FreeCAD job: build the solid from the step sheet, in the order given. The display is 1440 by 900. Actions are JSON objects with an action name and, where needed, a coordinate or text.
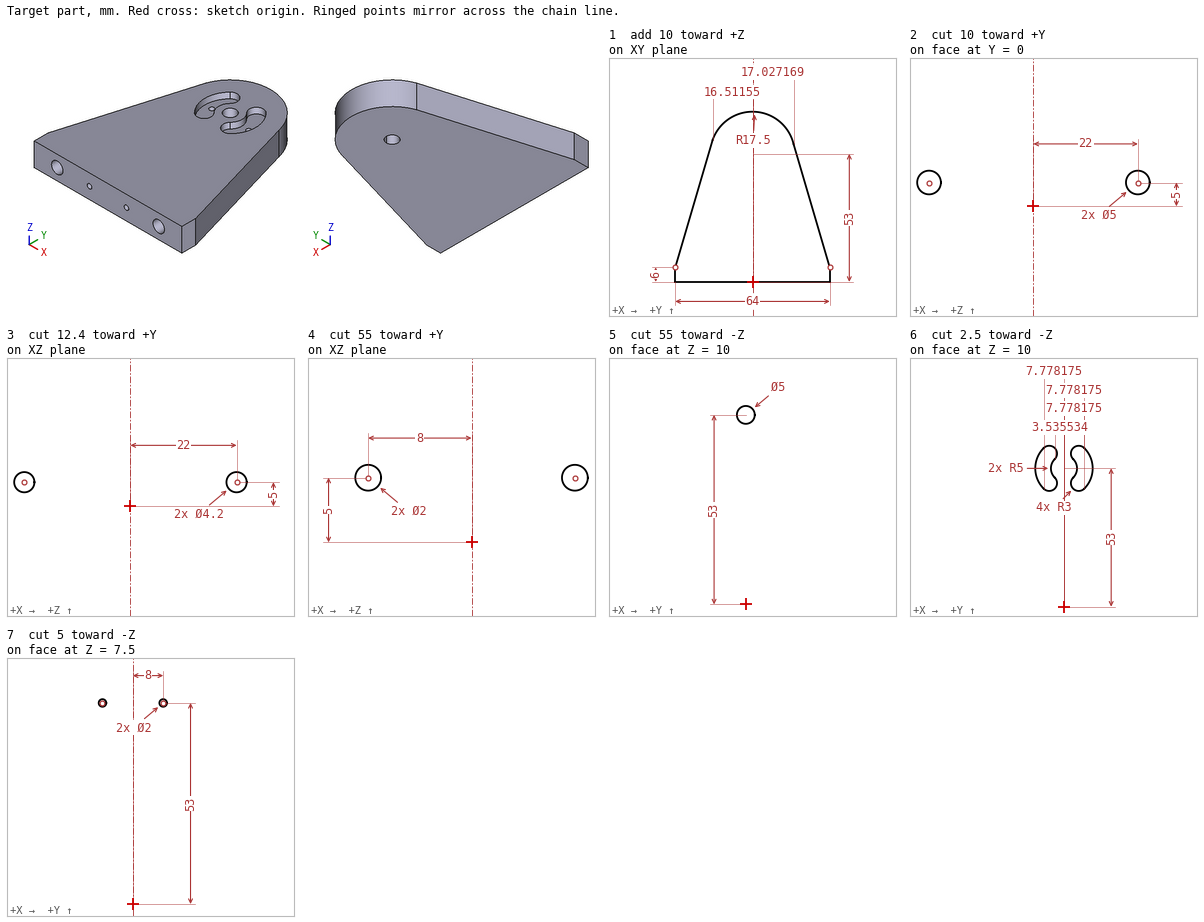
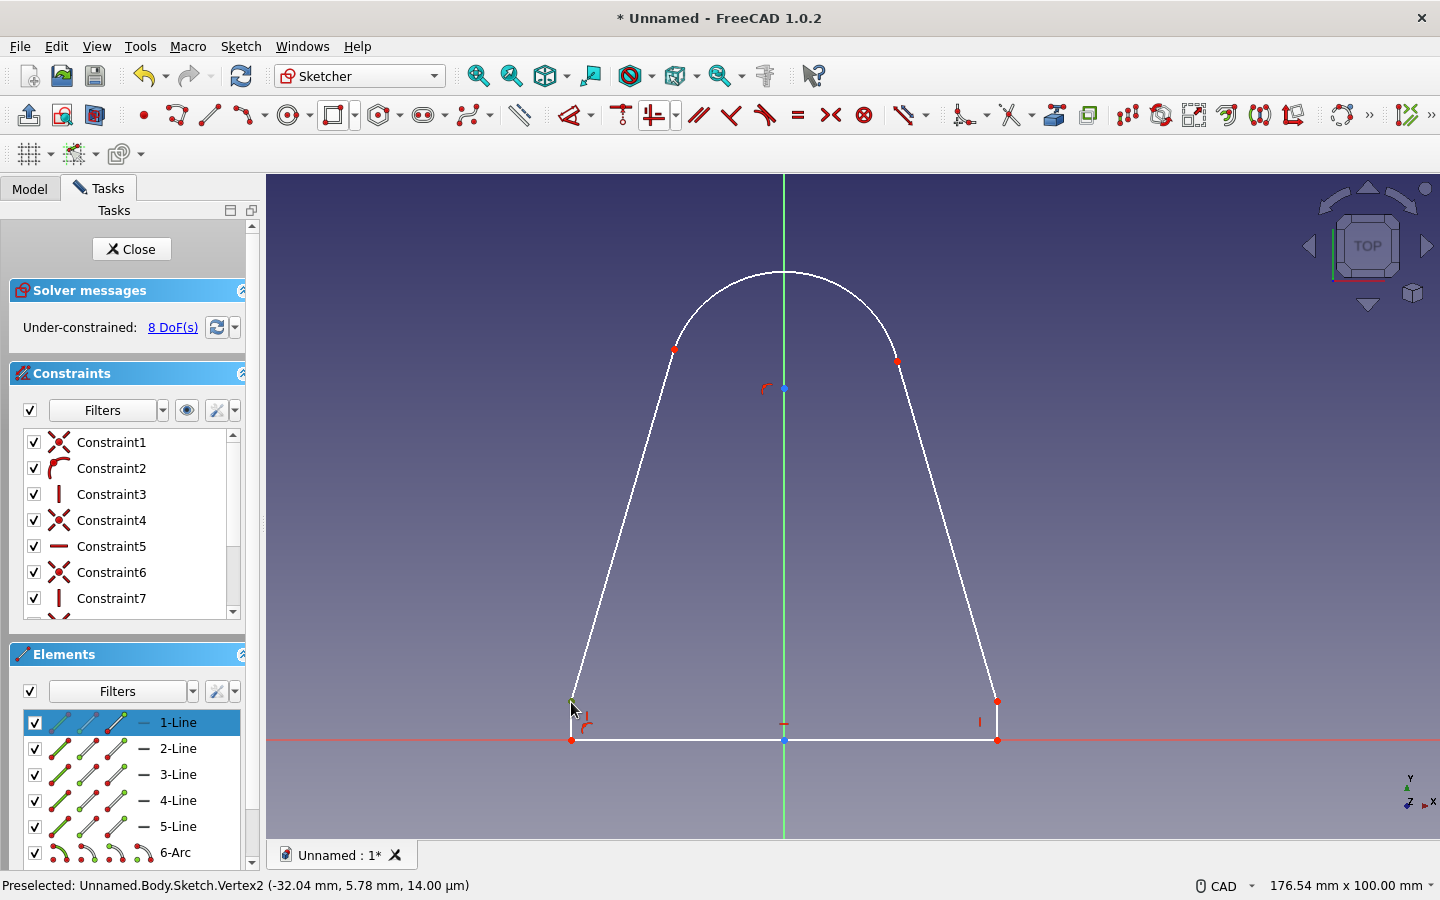
{"action": "left_click", "coordinate": [997, 702]}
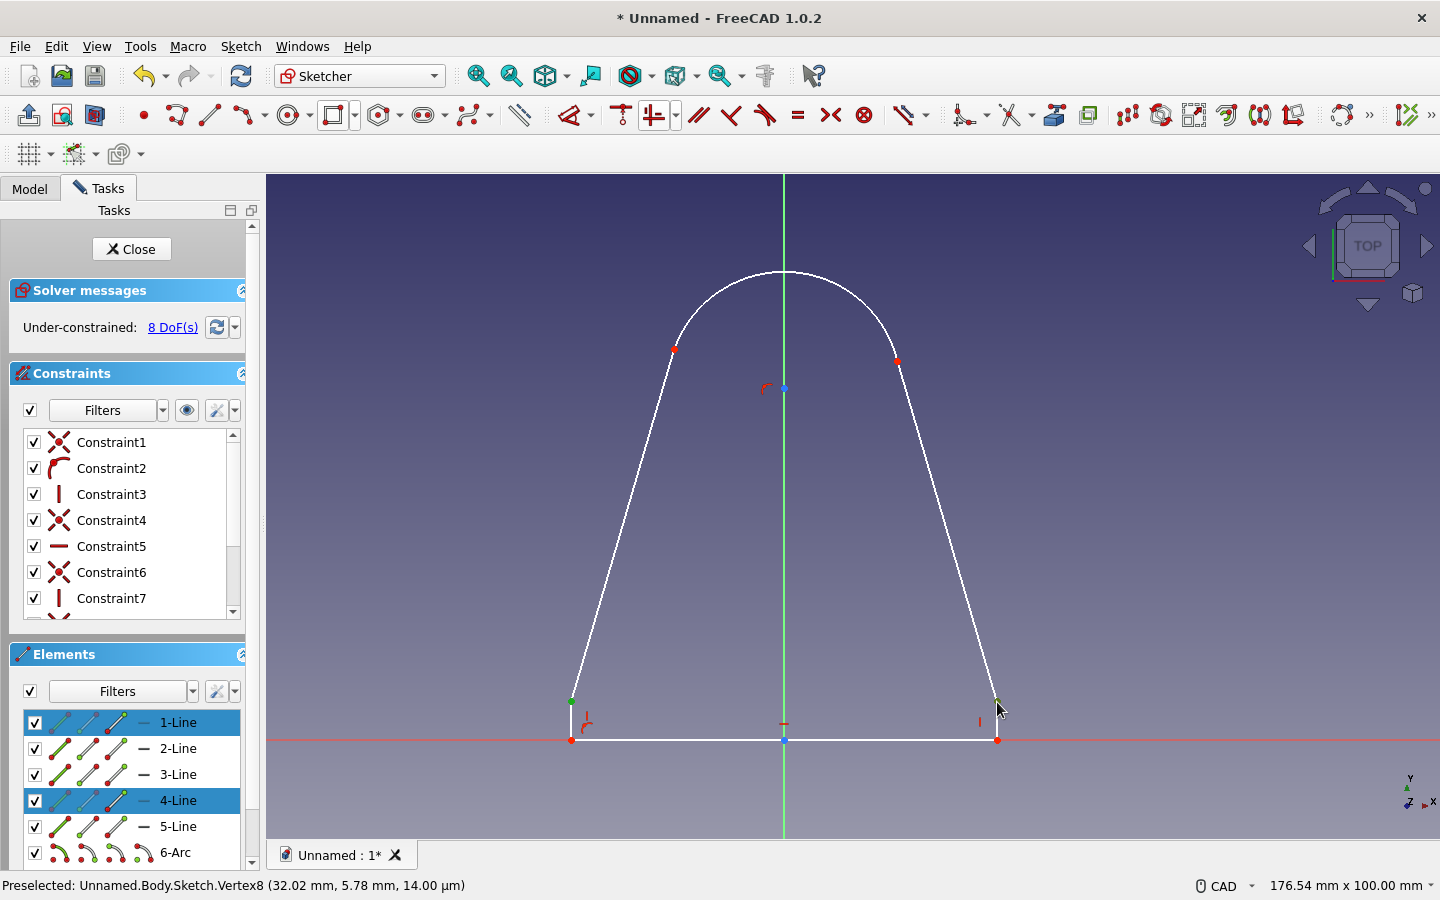
{"action": "left_click", "coordinate": [784, 680]}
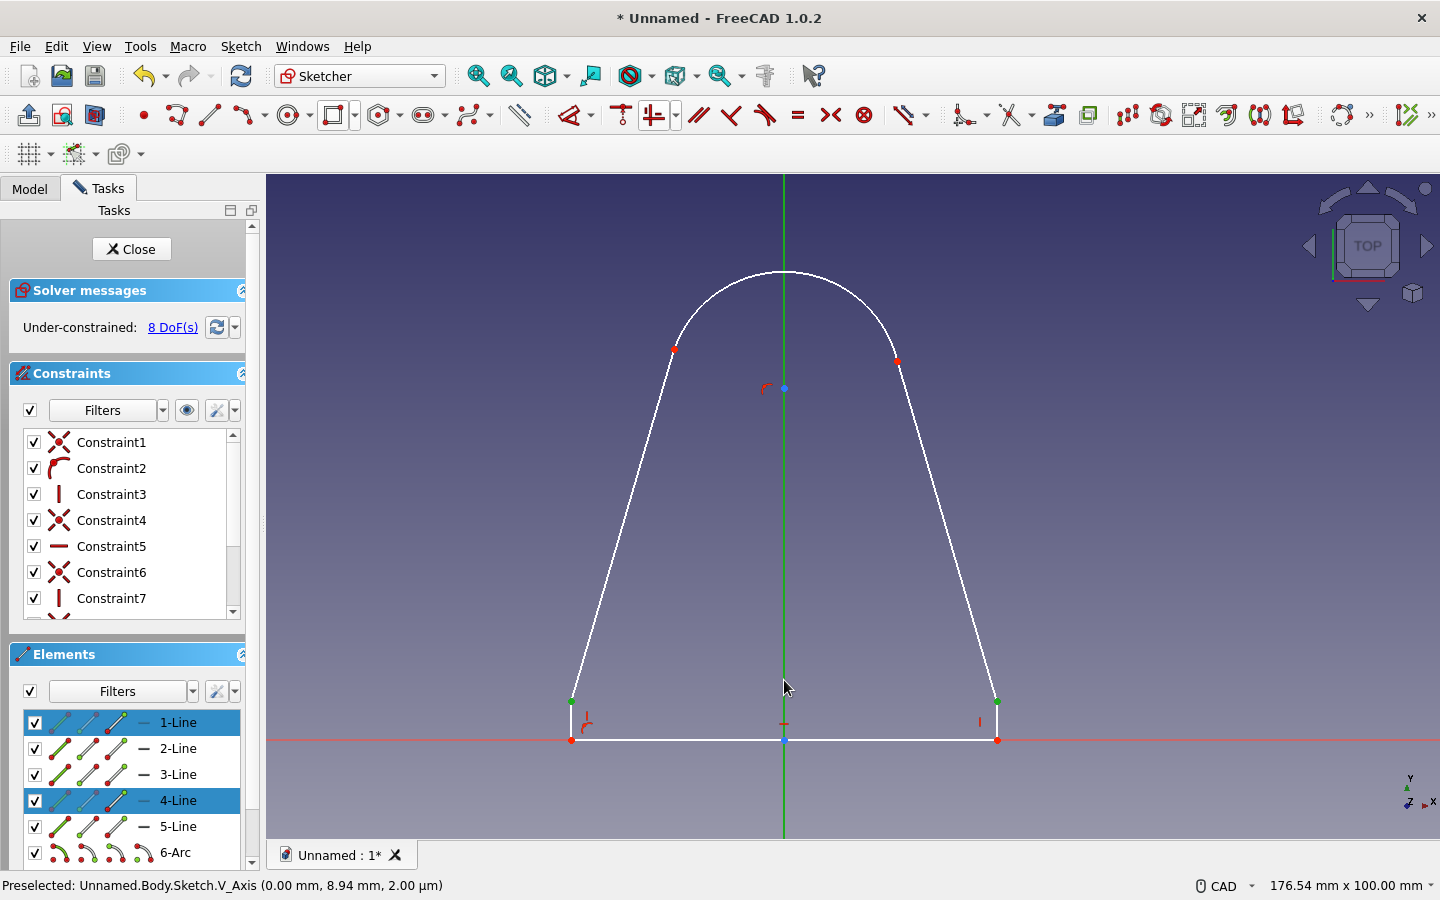
{"action": "left_click", "coordinate": [831, 116]}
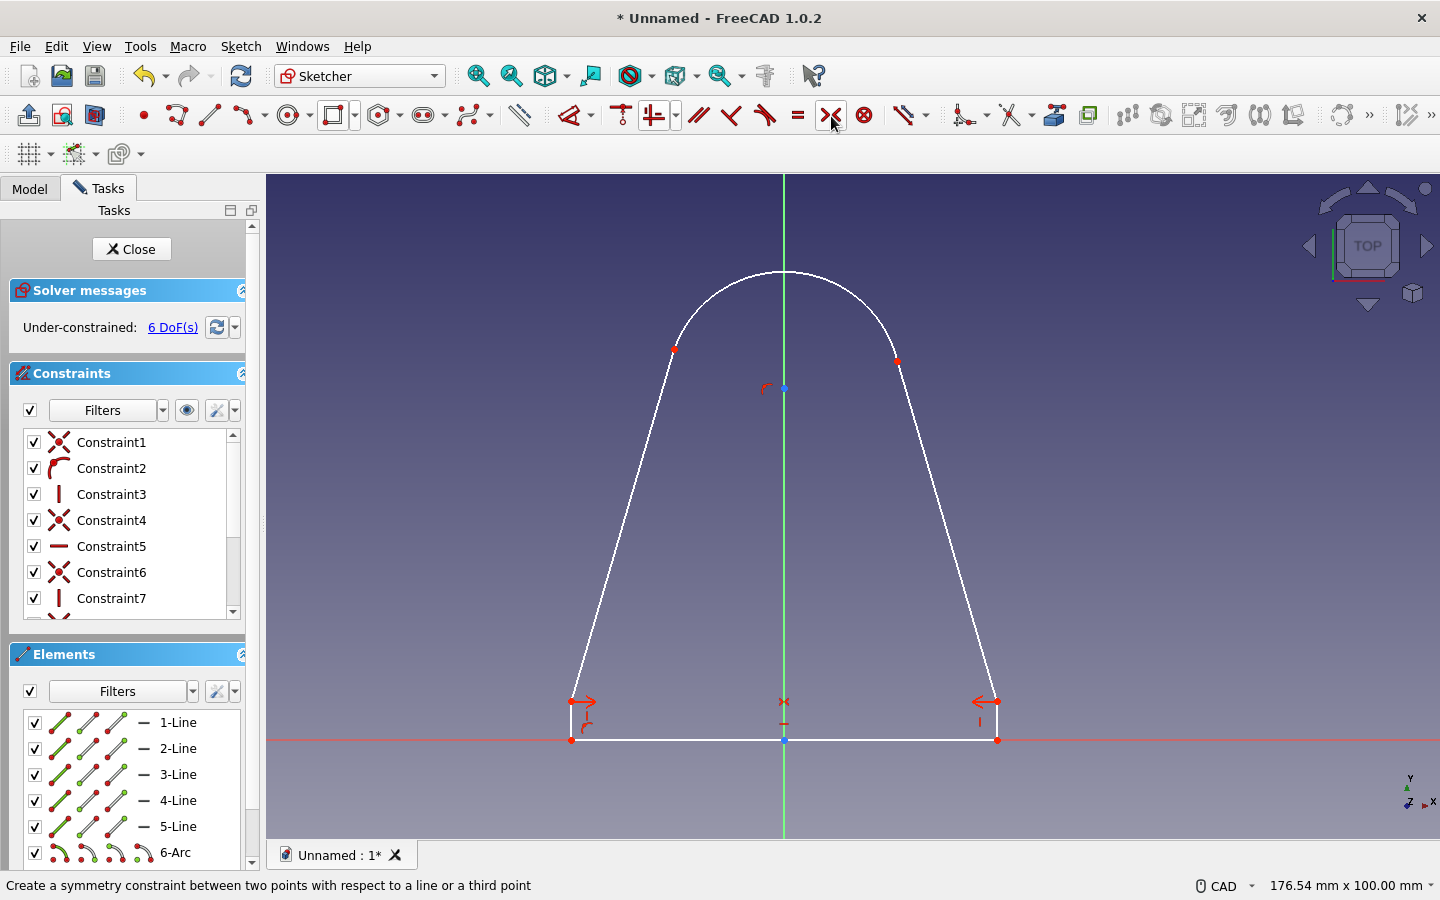
{"action": "left_click", "coordinate": [568, 116]}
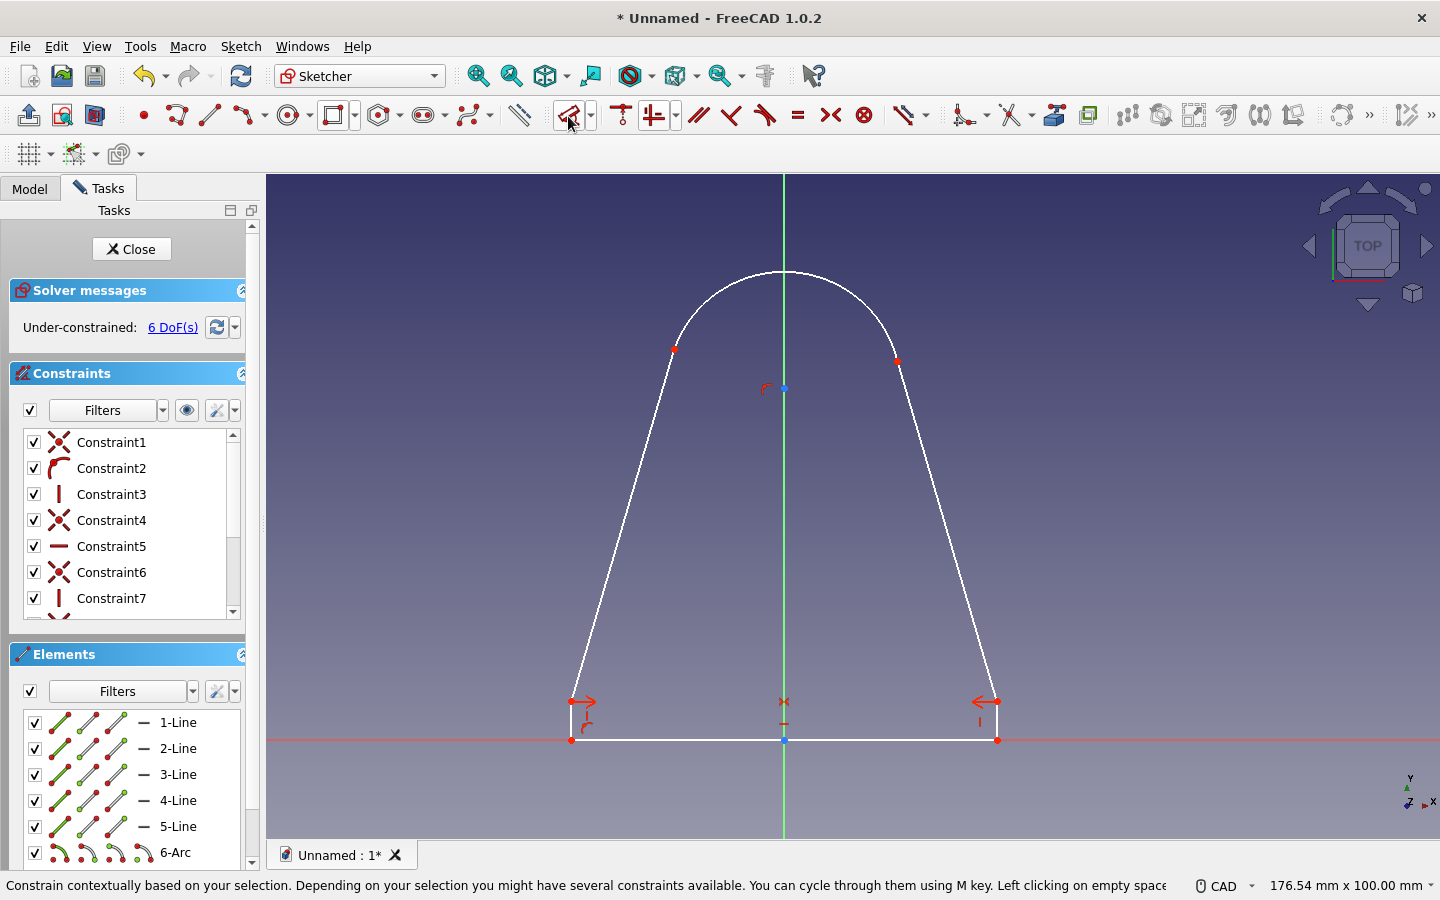
{"action": "left_click", "coordinate": [847, 290]}
{"action": "left_click", "coordinate": [864, 263]}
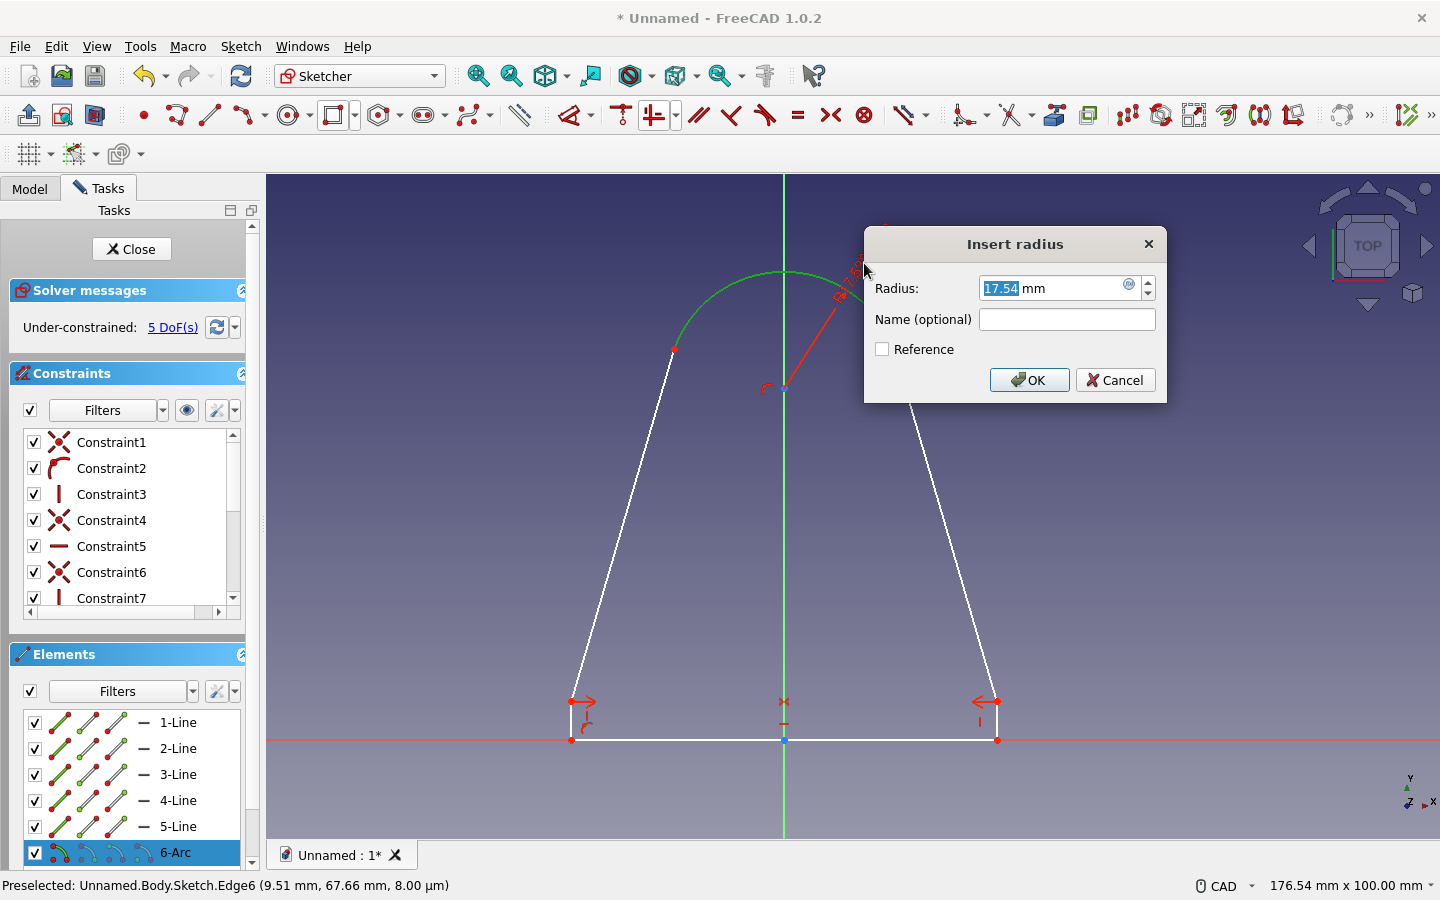
{"action": "type", "text": "17.5"}
{"action": "key", "text": "Return"}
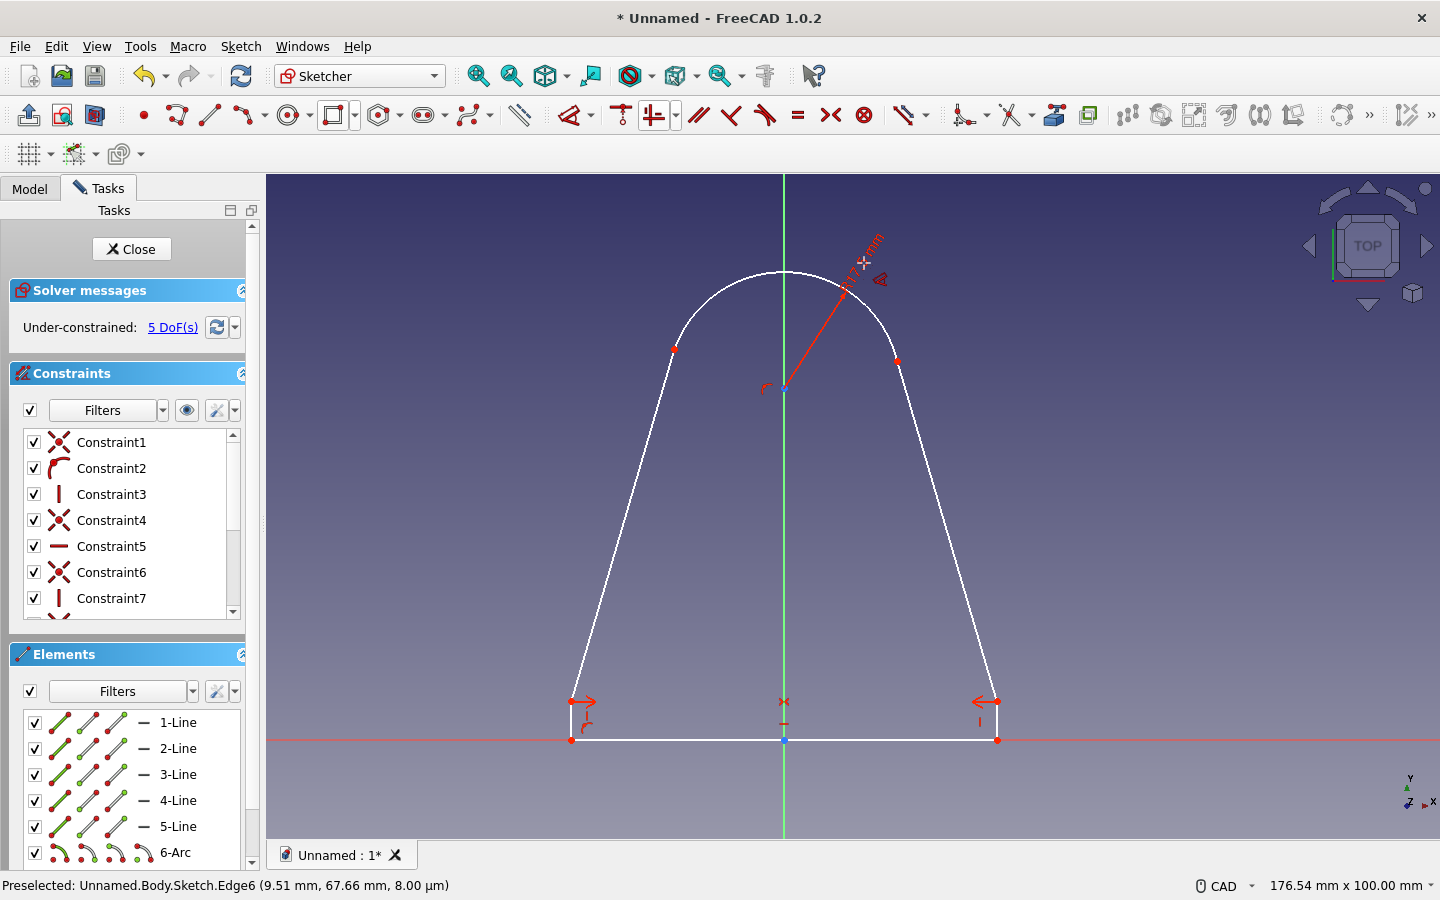
{"action": "left_click", "coordinate": [571, 714]}
{"action": "left_click", "coordinate": [537, 721]}